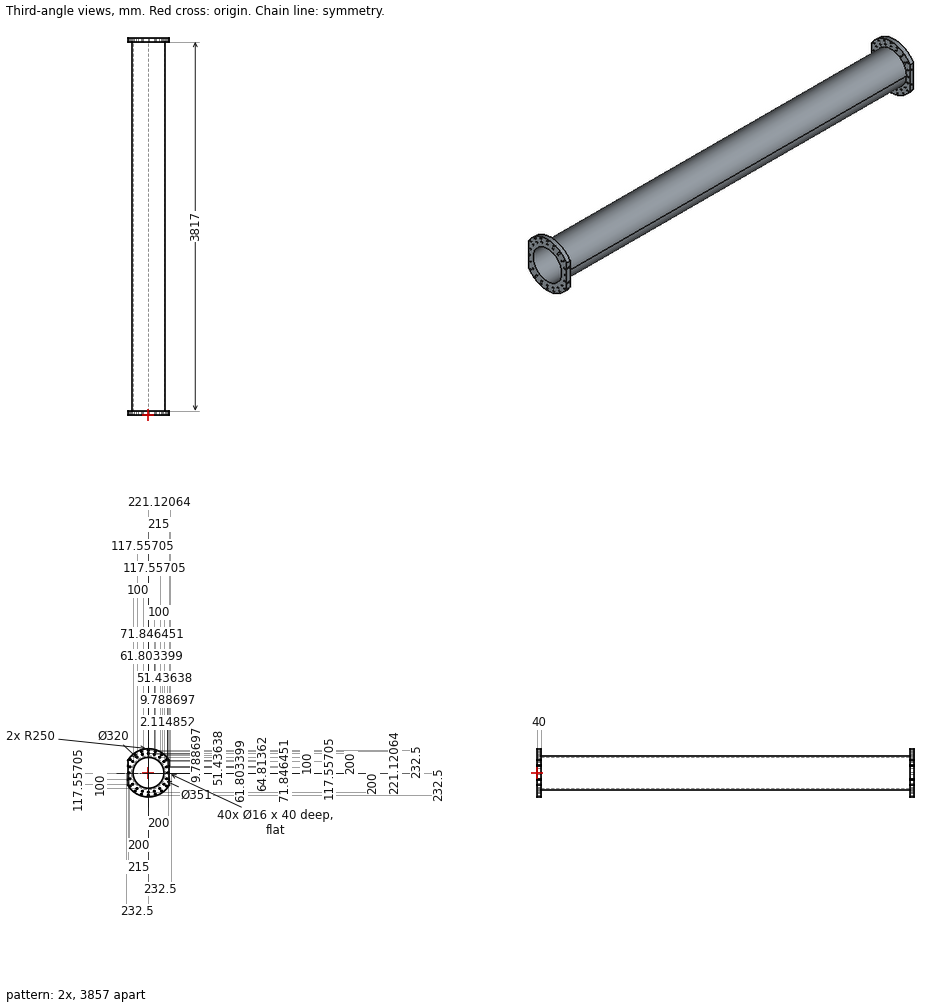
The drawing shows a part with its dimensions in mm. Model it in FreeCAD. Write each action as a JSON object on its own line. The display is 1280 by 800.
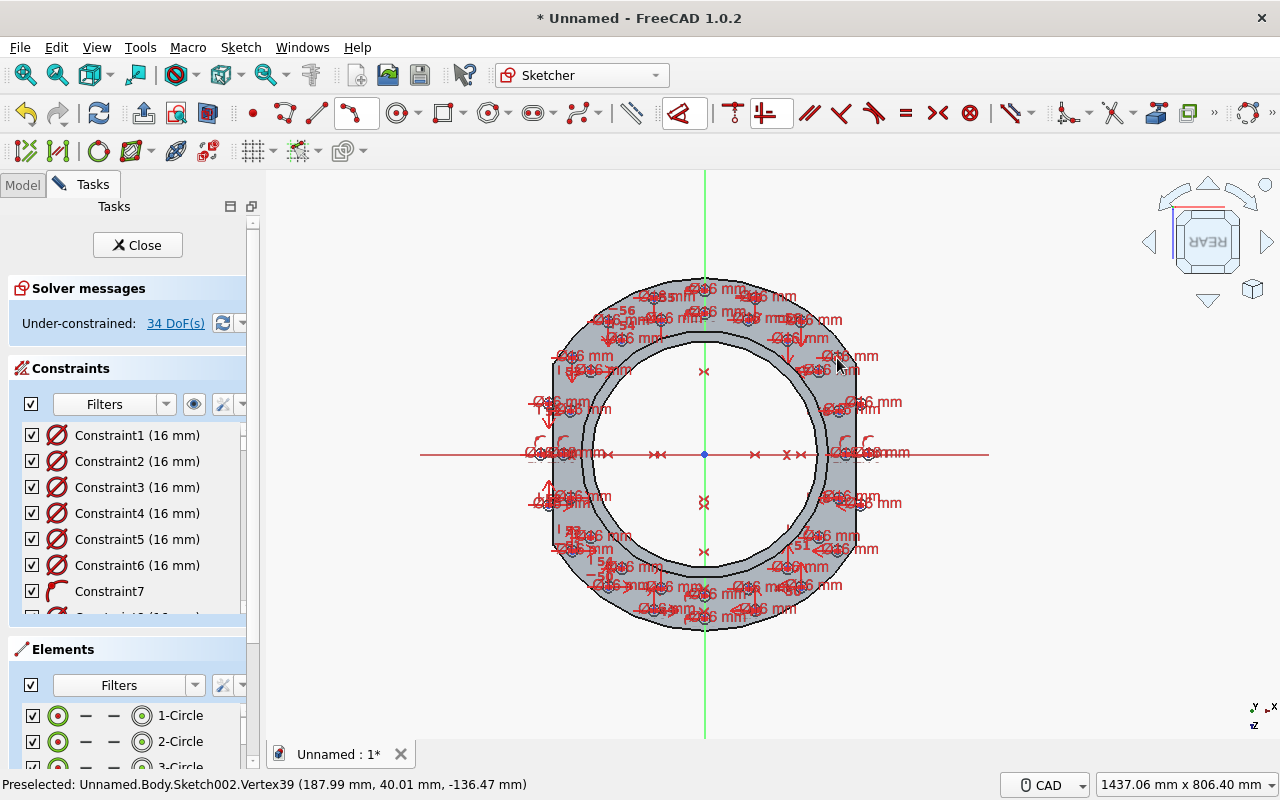
{"action": "left_click", "coordinate": [470, 454]}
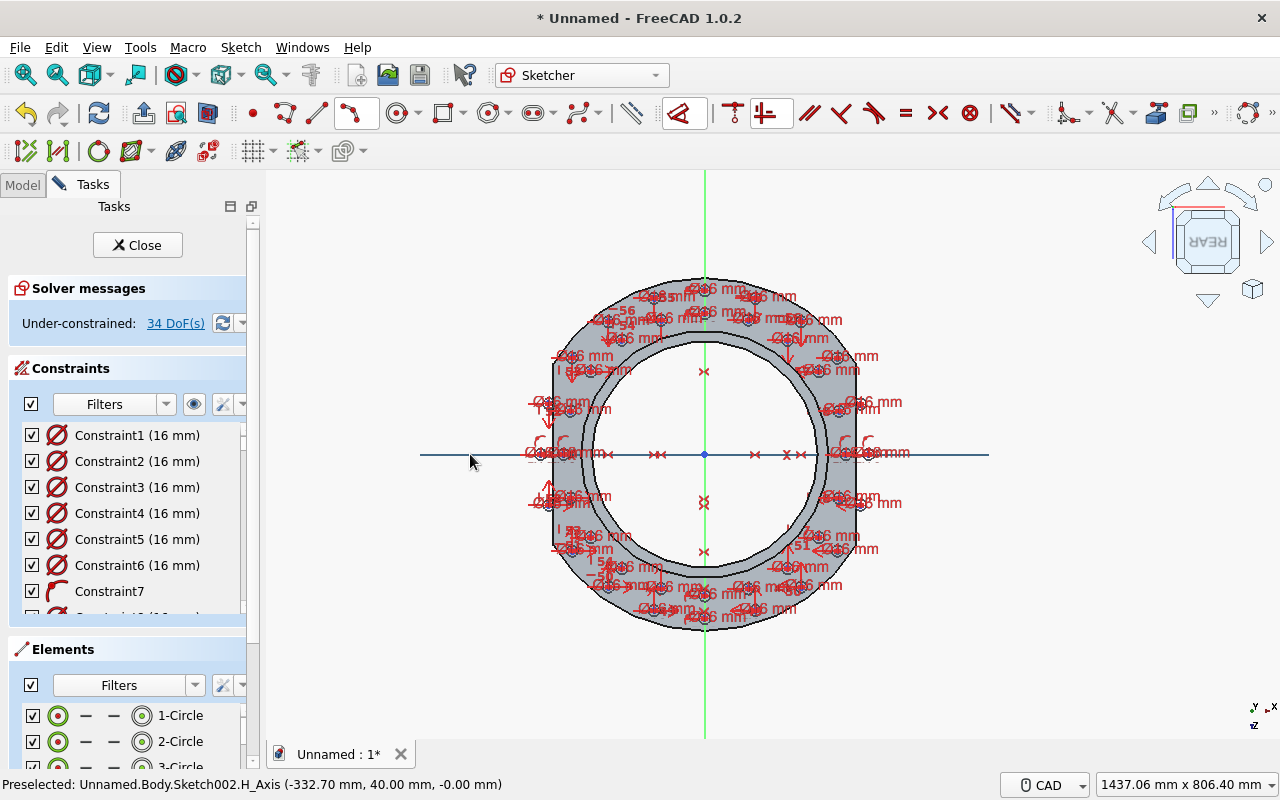
{"action": "left_click", "coordinate": [938, 114]}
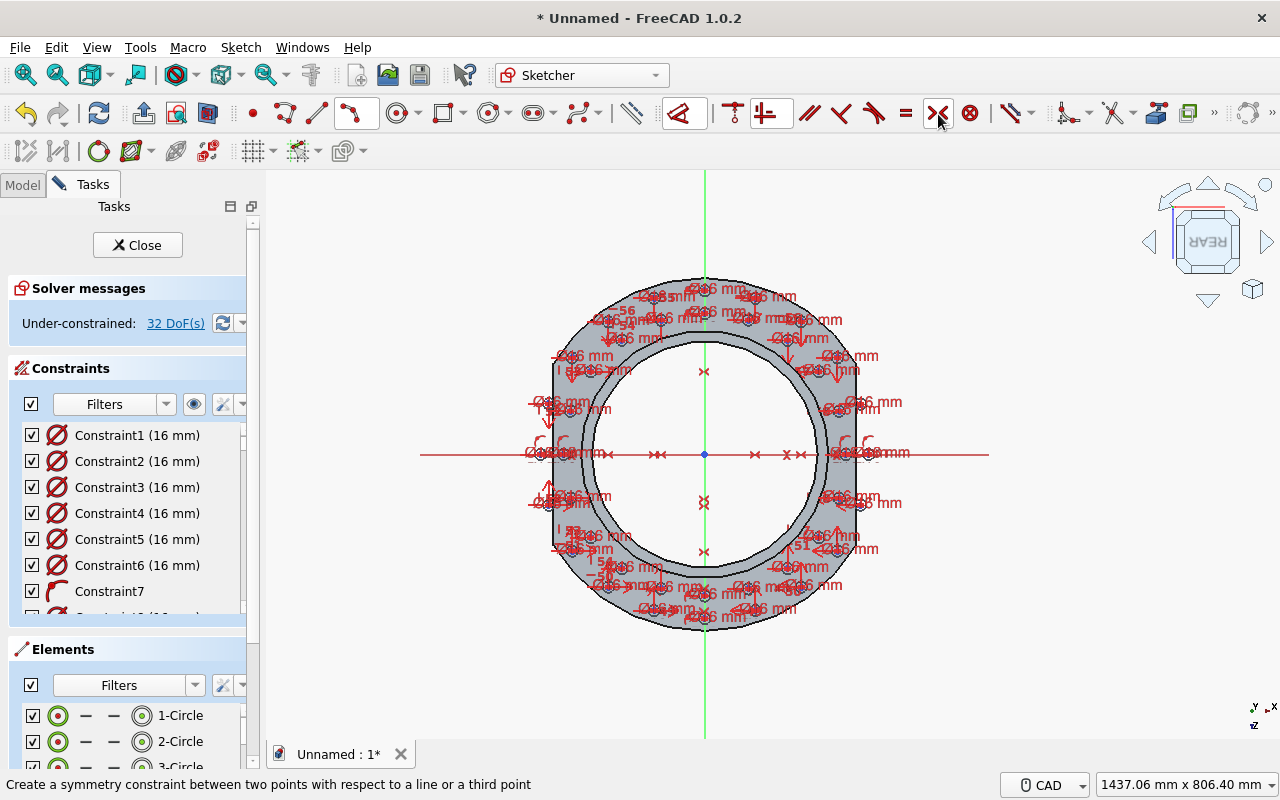
{"action": "left_click", "coordinate": [861, 505]}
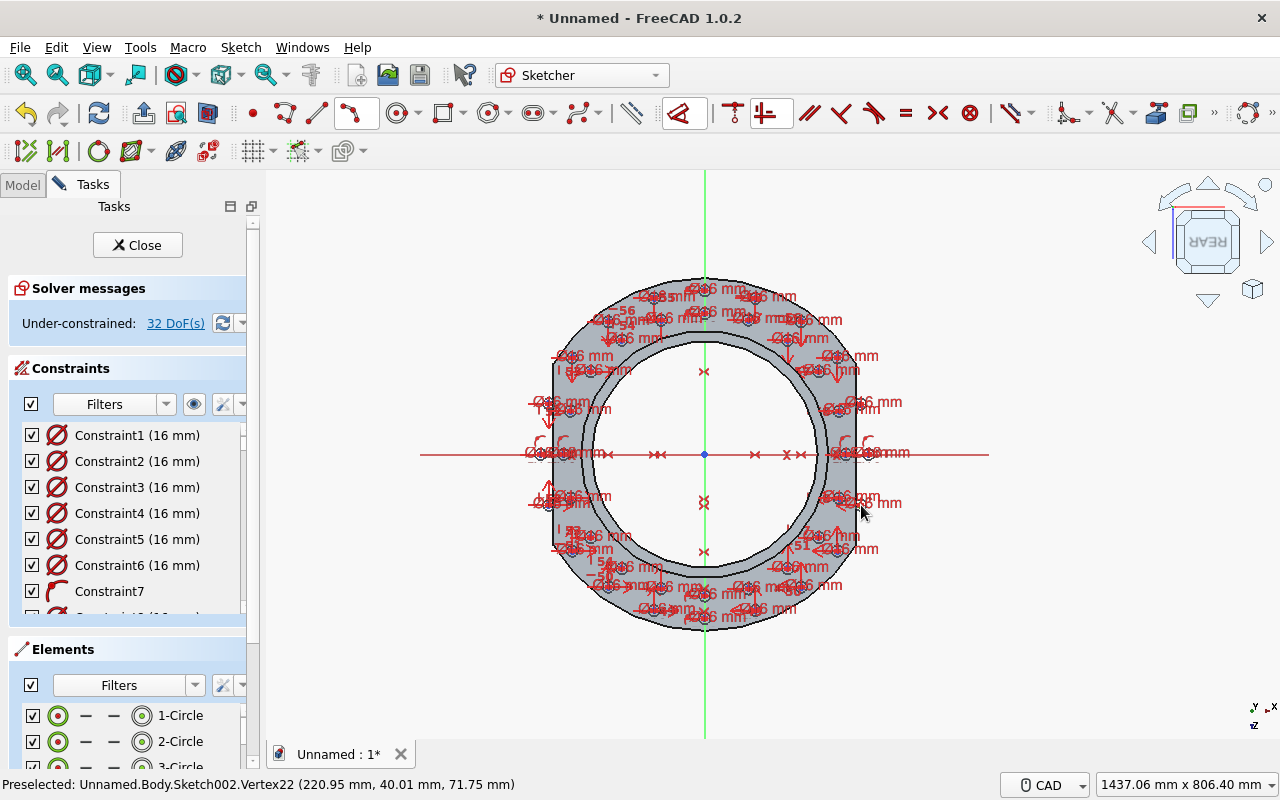
{"action": "left_click", "coordinate": [861, 404]}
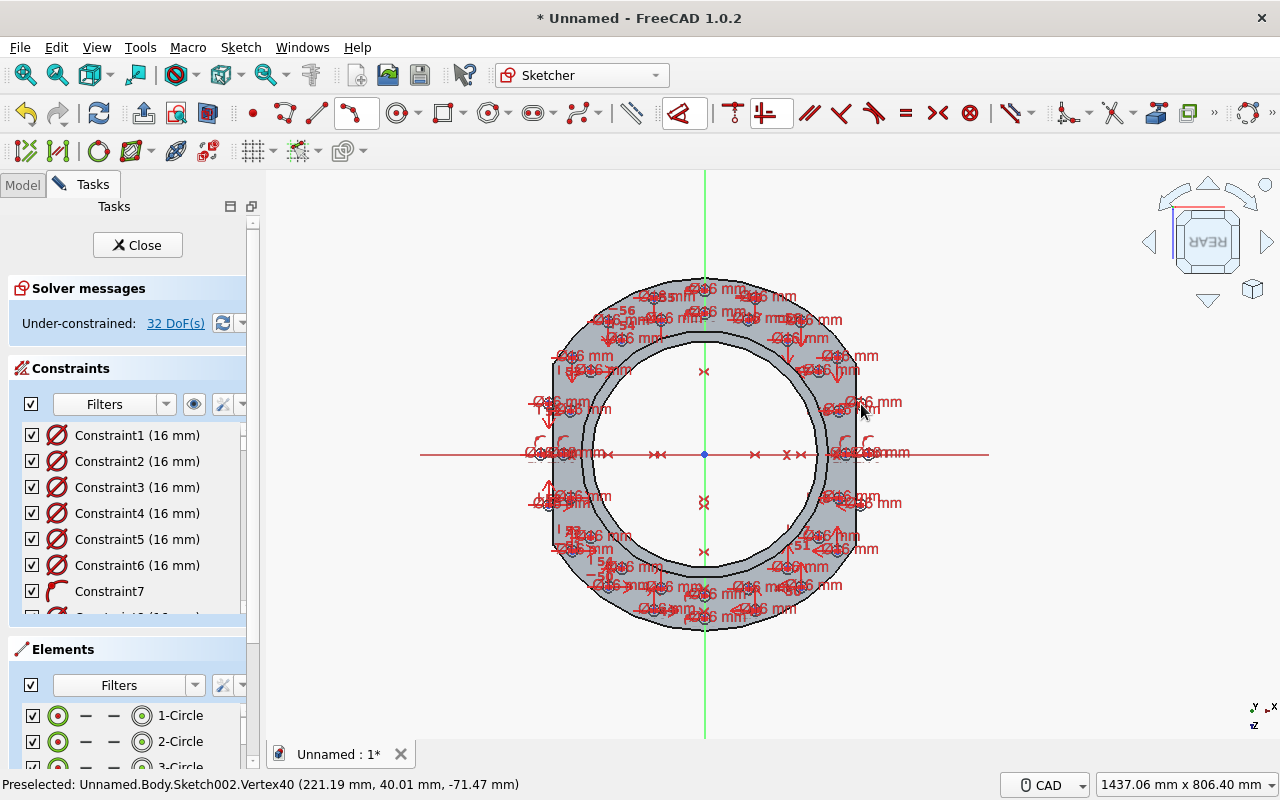
{"action": "left_click", "coordinate": [470, 454]}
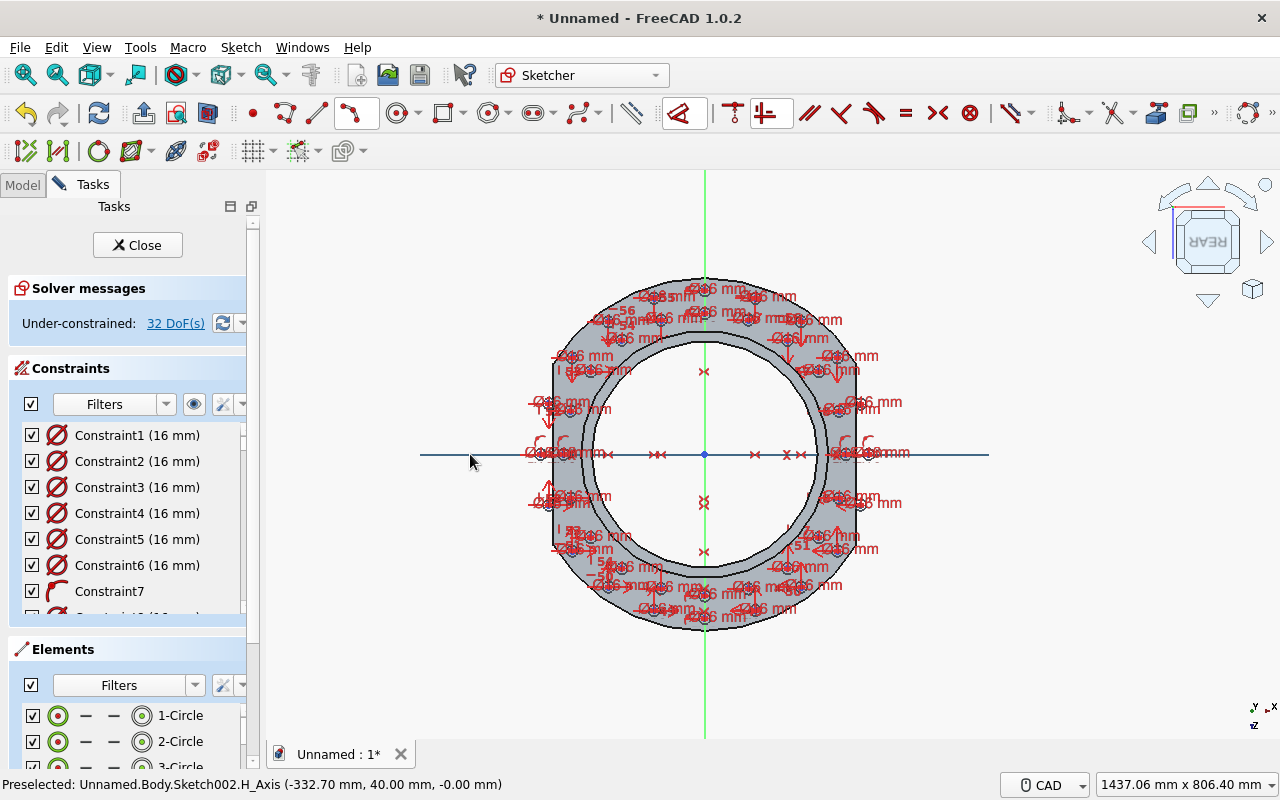
{"action": "left_click", "coordinate": [938, 114]}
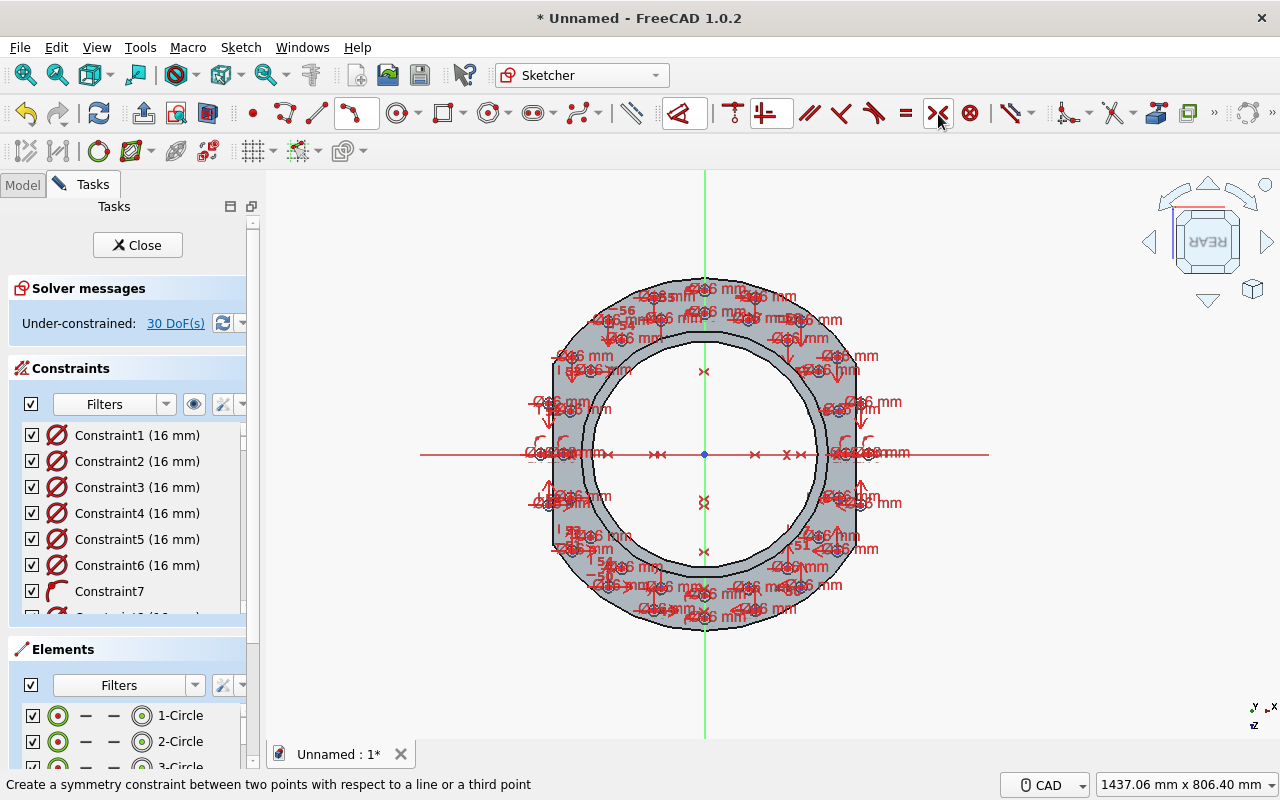
{"action": "left_click", "coordinate": [846, 454]}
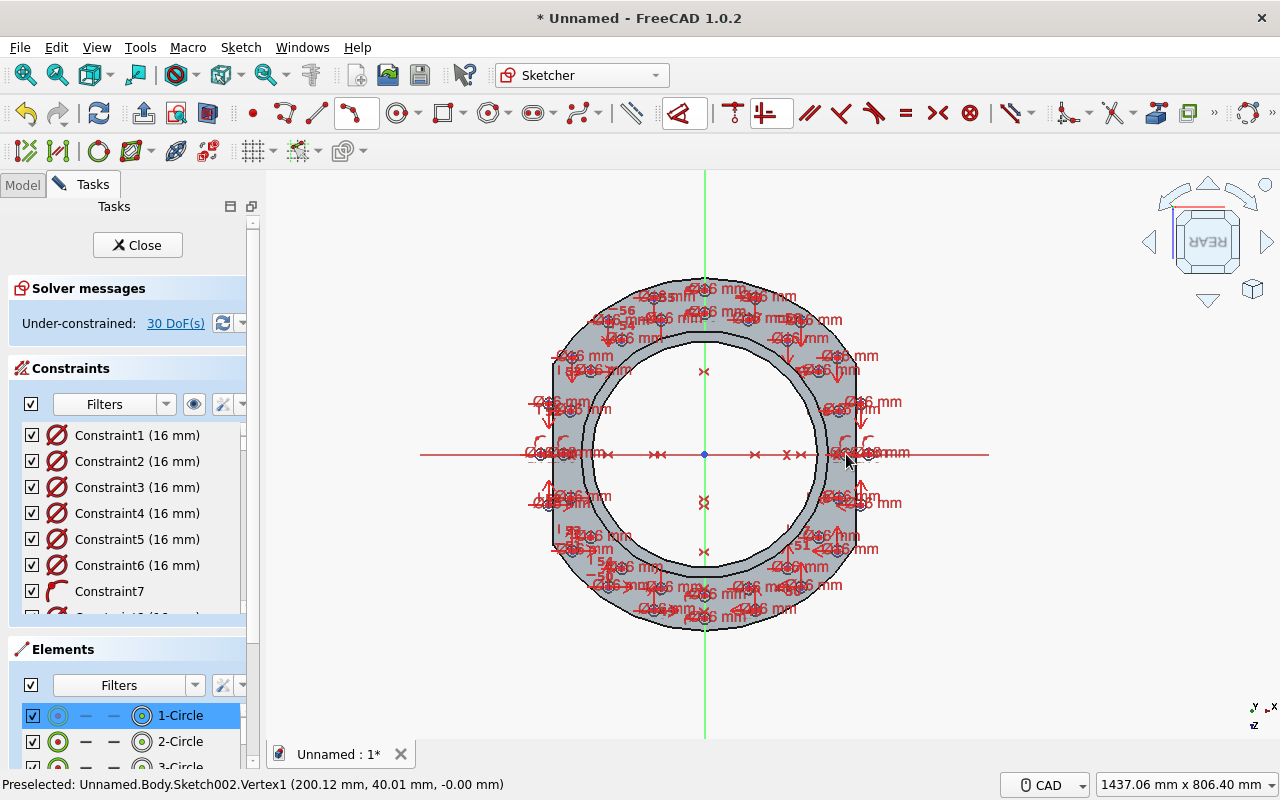
{"action": "key", "text": "l"}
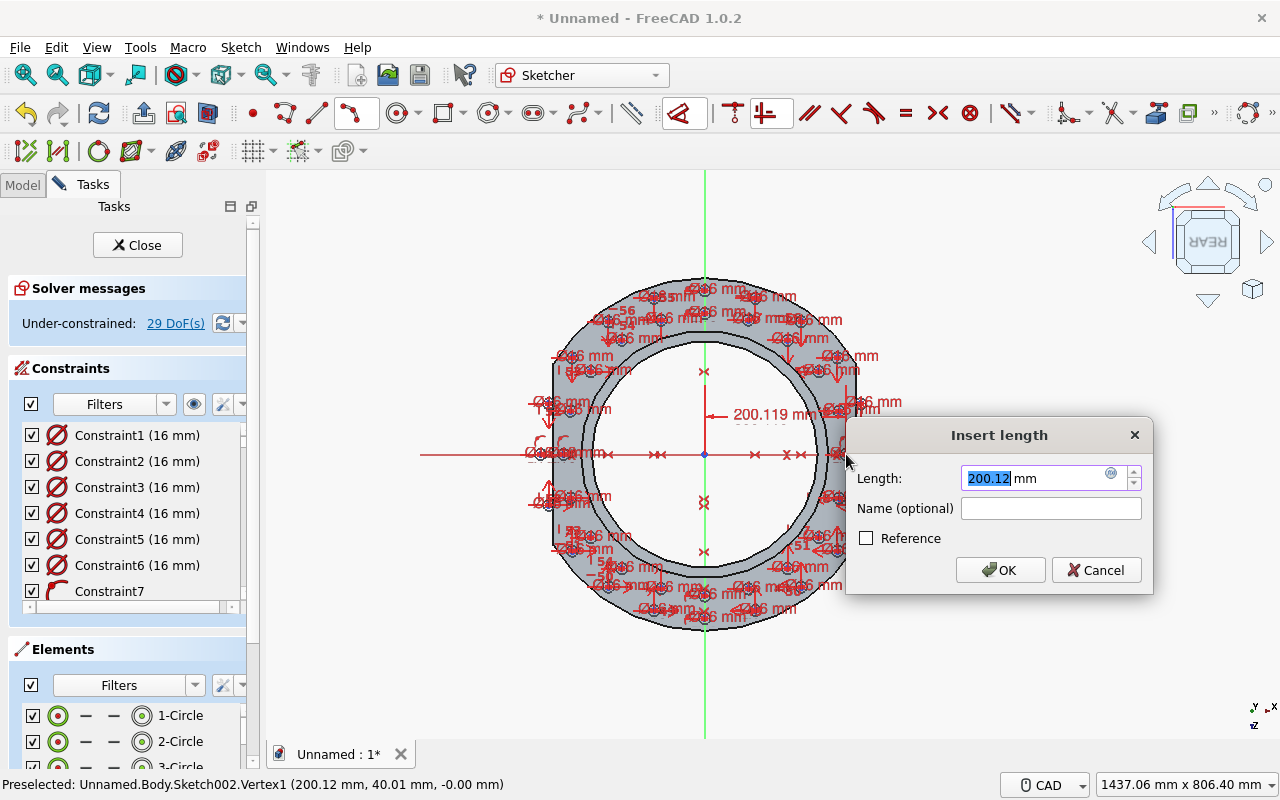
{"action": "type", "text": "200"}
{"action": "key", "text": "Return"}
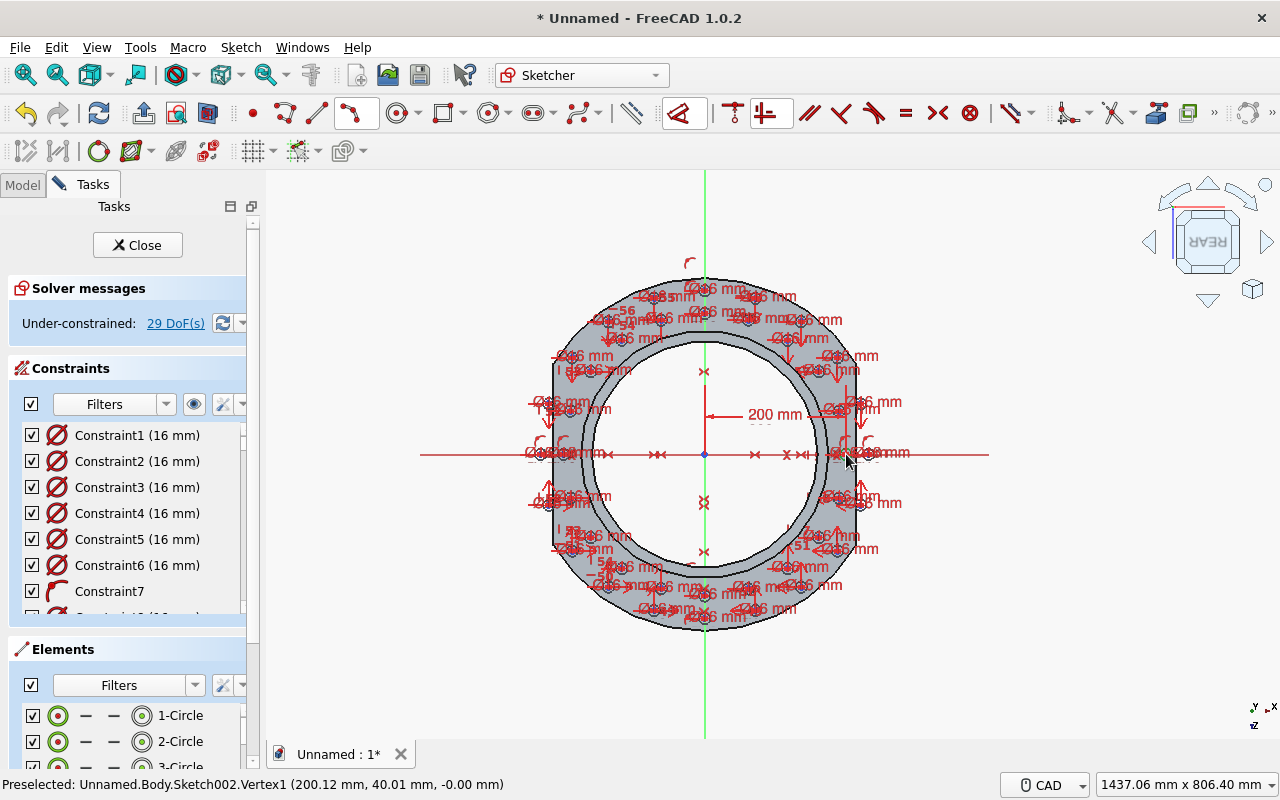
{"action": "left_click", "coordinate": [705, 596]}